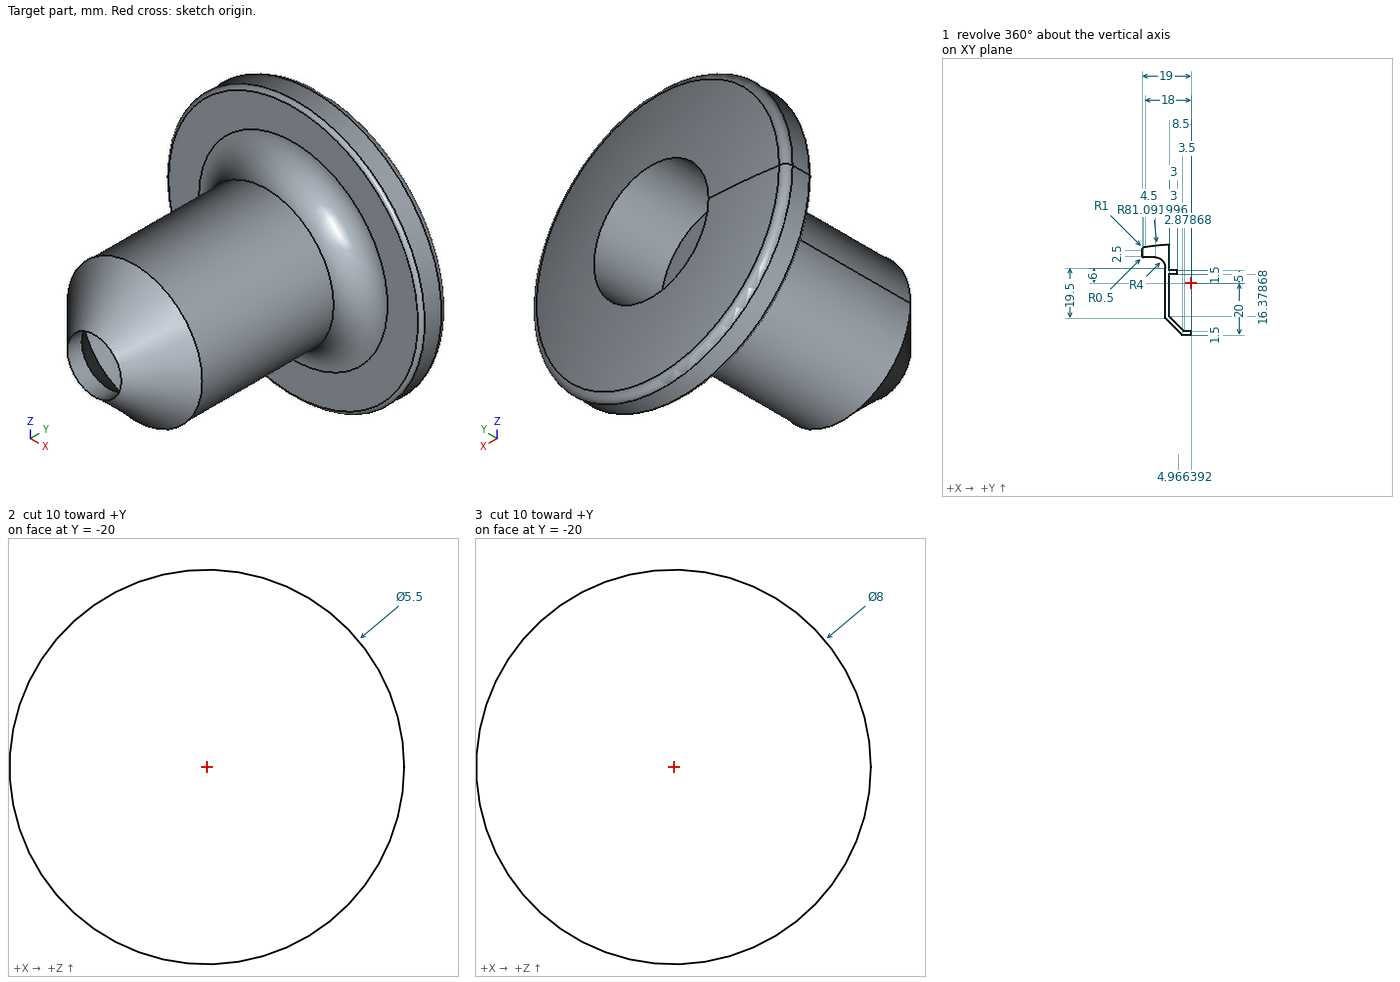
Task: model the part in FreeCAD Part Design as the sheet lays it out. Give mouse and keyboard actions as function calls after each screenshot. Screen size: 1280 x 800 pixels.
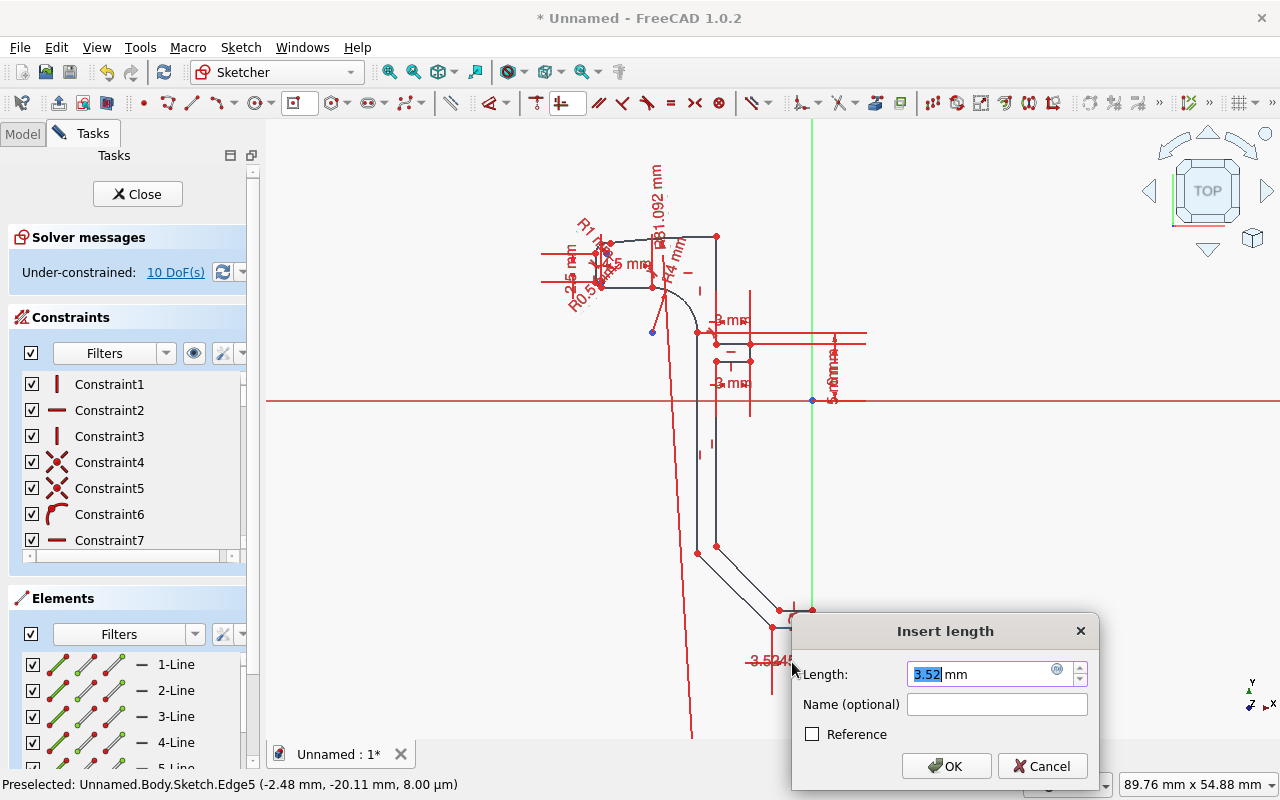
text(3.5)
key(Return)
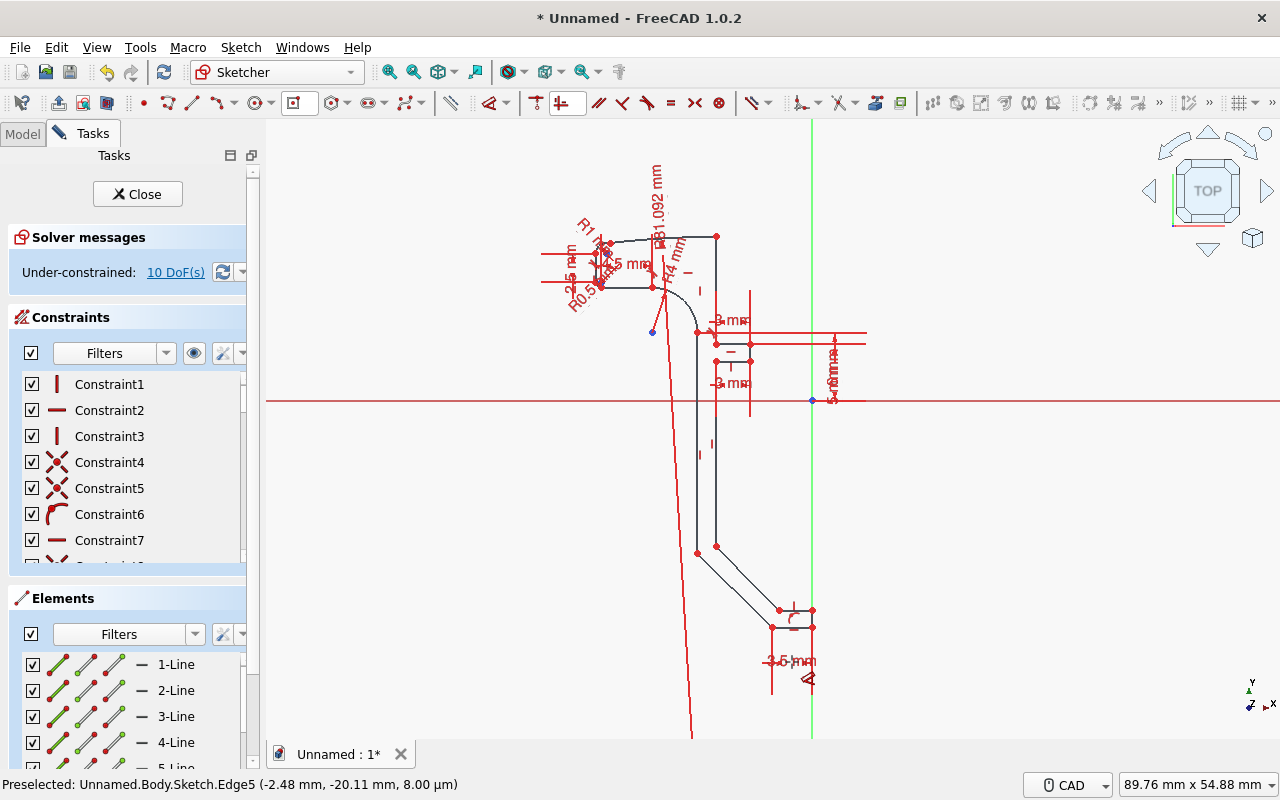
scroll(812, 619, up, 5)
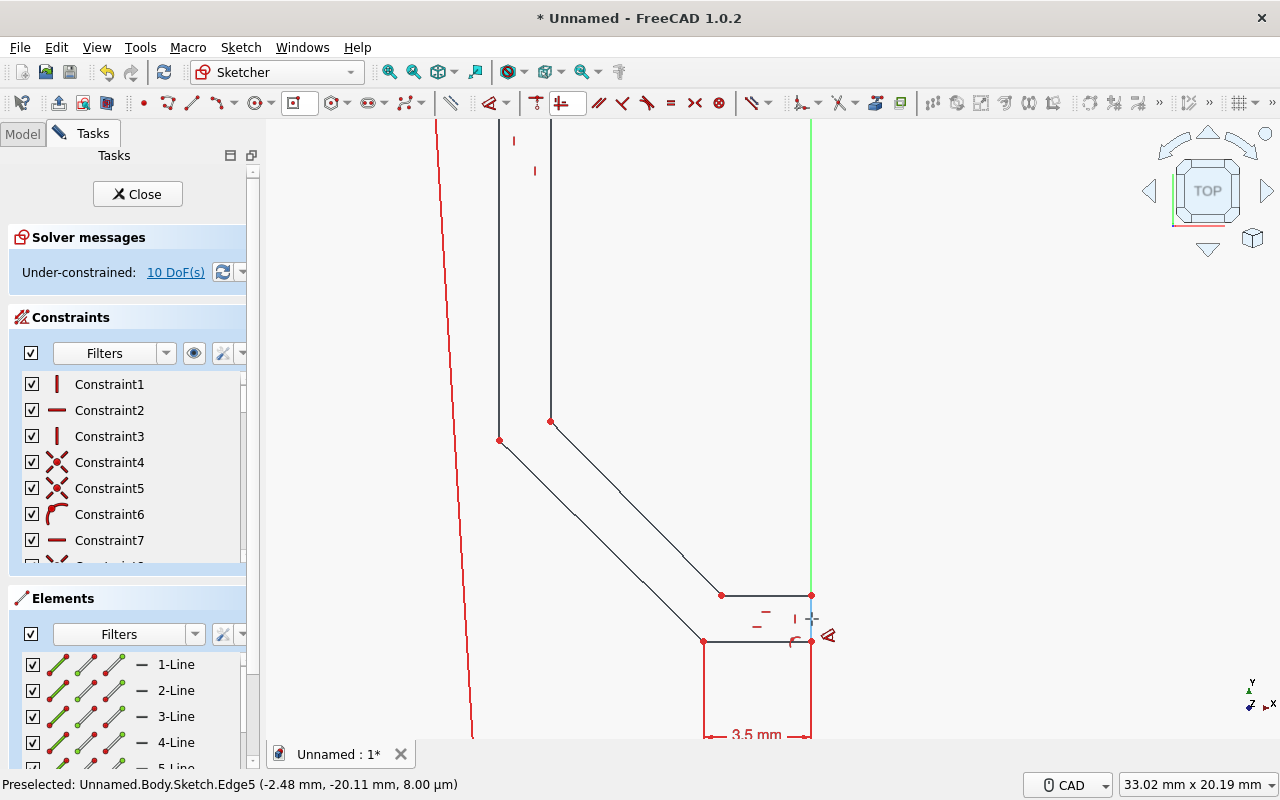
click(811, 619)
click(845, 619)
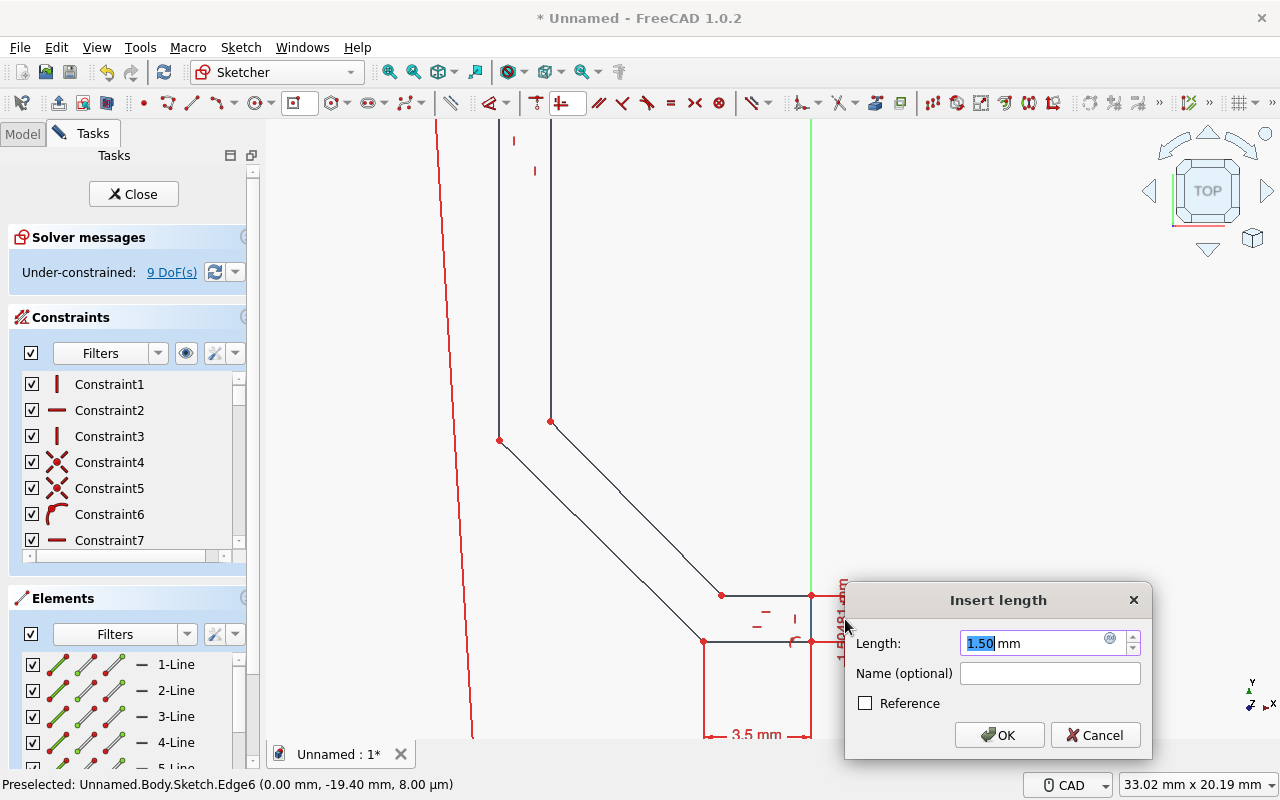
text(1.5)
key(Return)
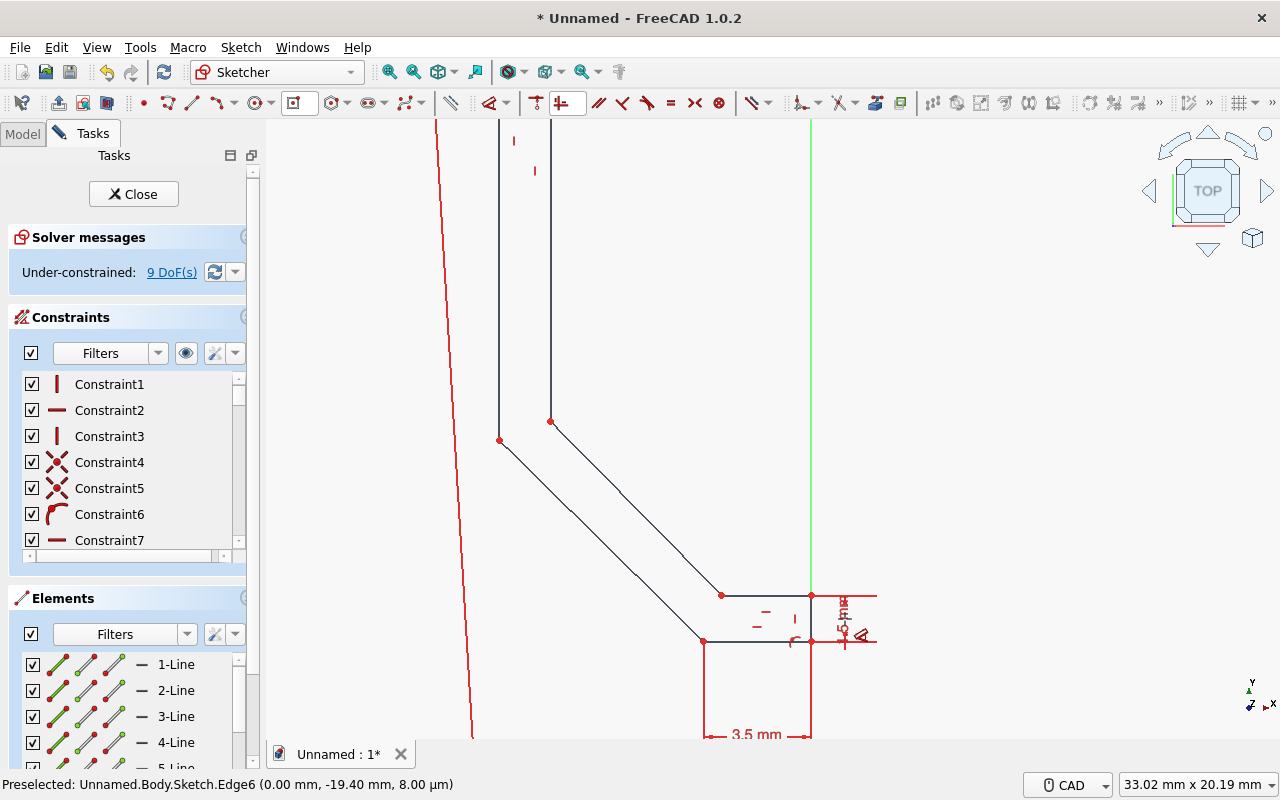
scroll(812, 620, down, 5)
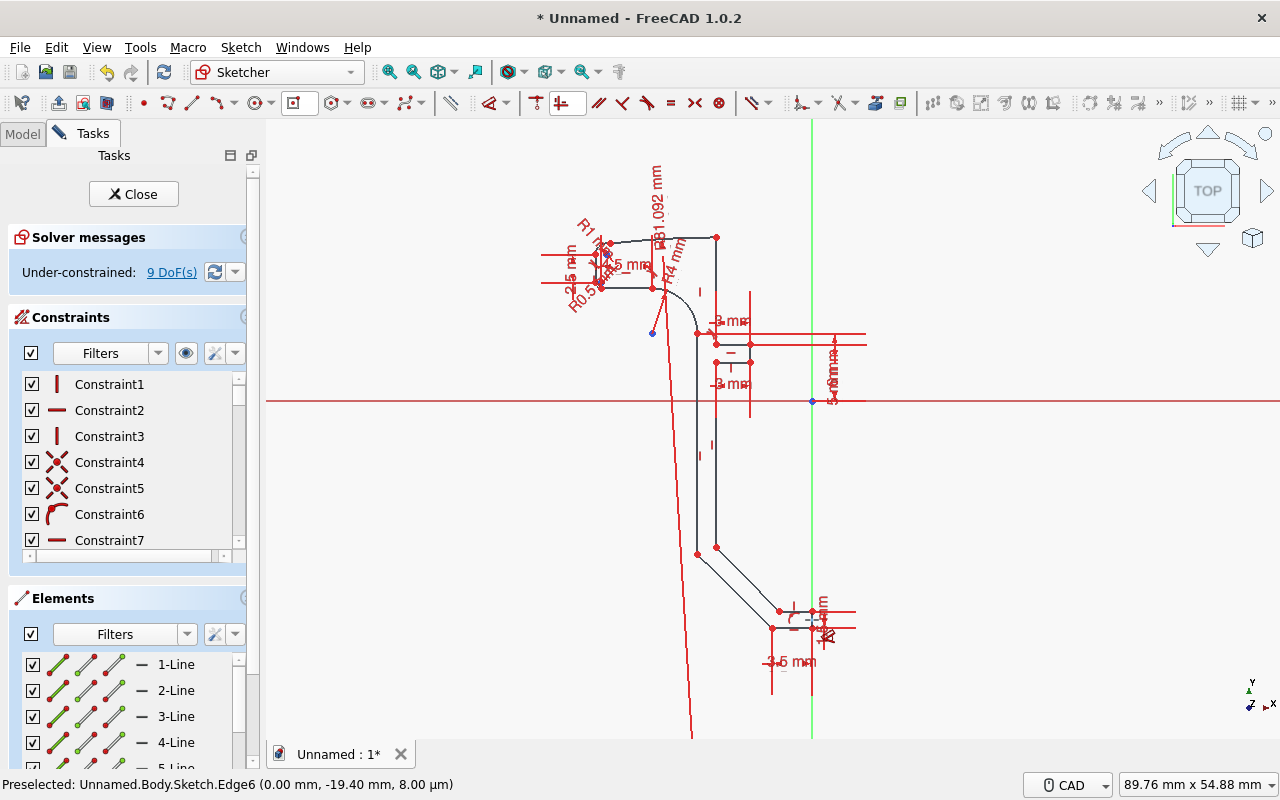
scroll(750, 357, up, 5)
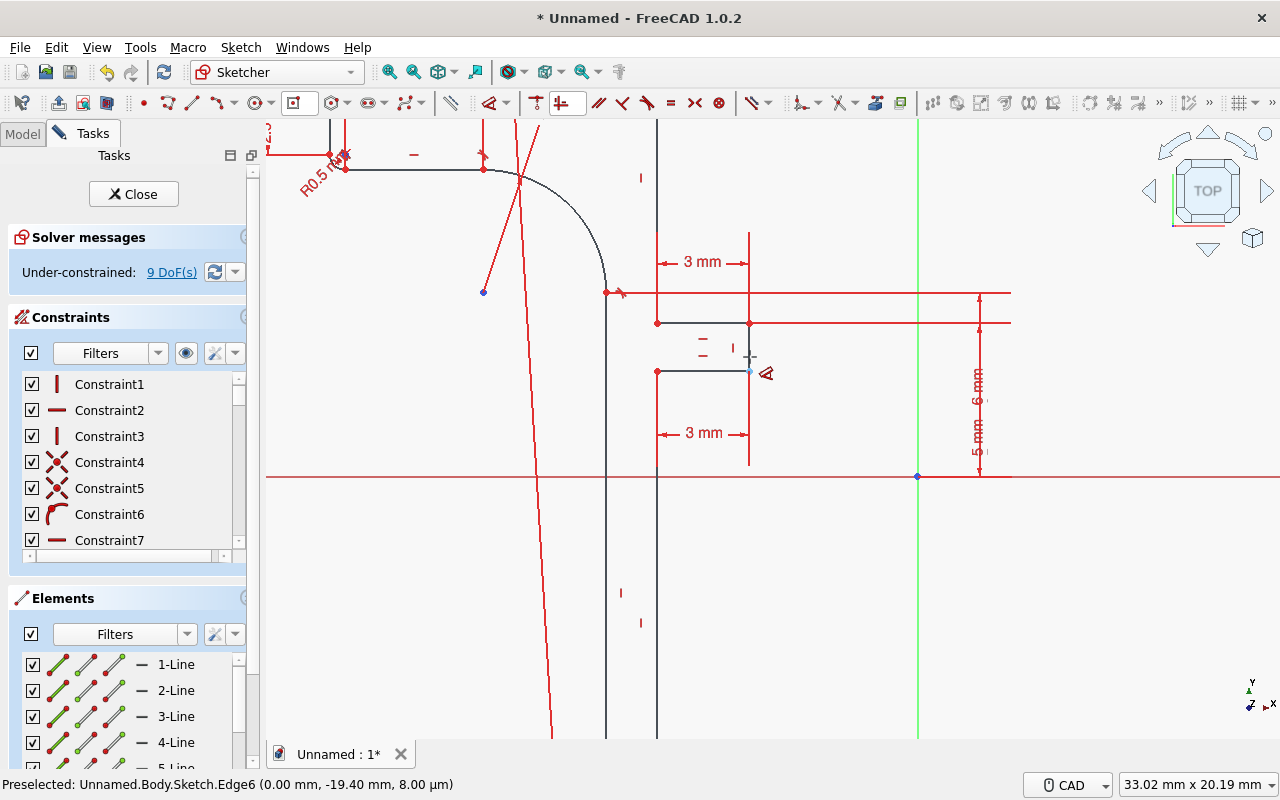
click(749, 357)
click(783, 347)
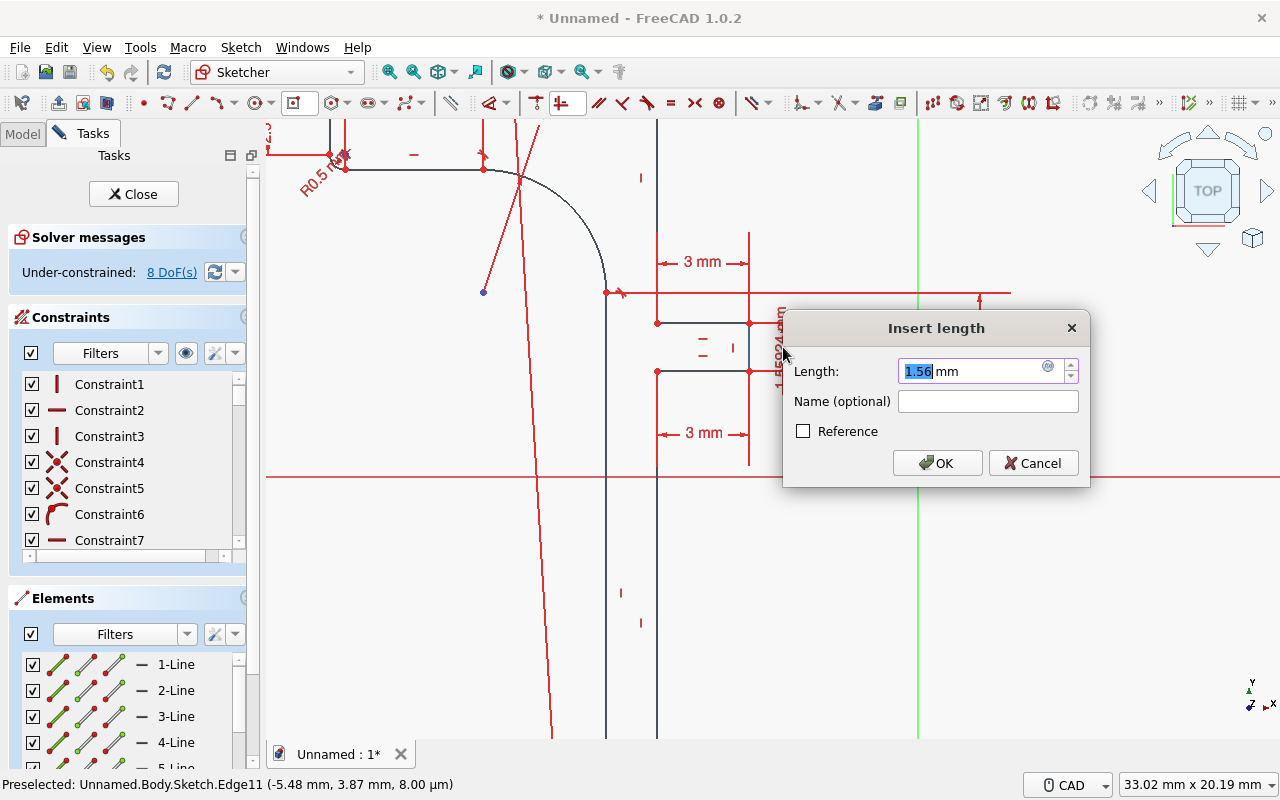
text(1.5)
key(Return)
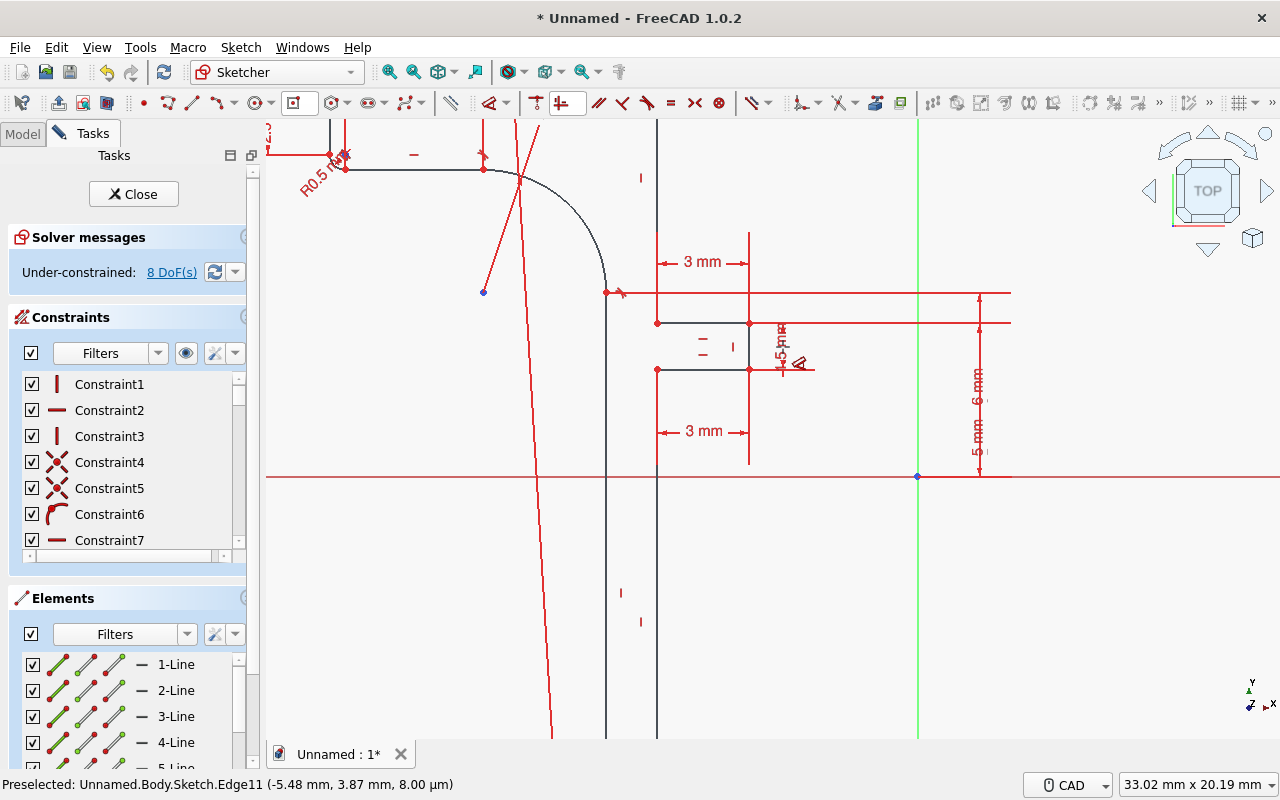
scroll(750, 356, down, 5)